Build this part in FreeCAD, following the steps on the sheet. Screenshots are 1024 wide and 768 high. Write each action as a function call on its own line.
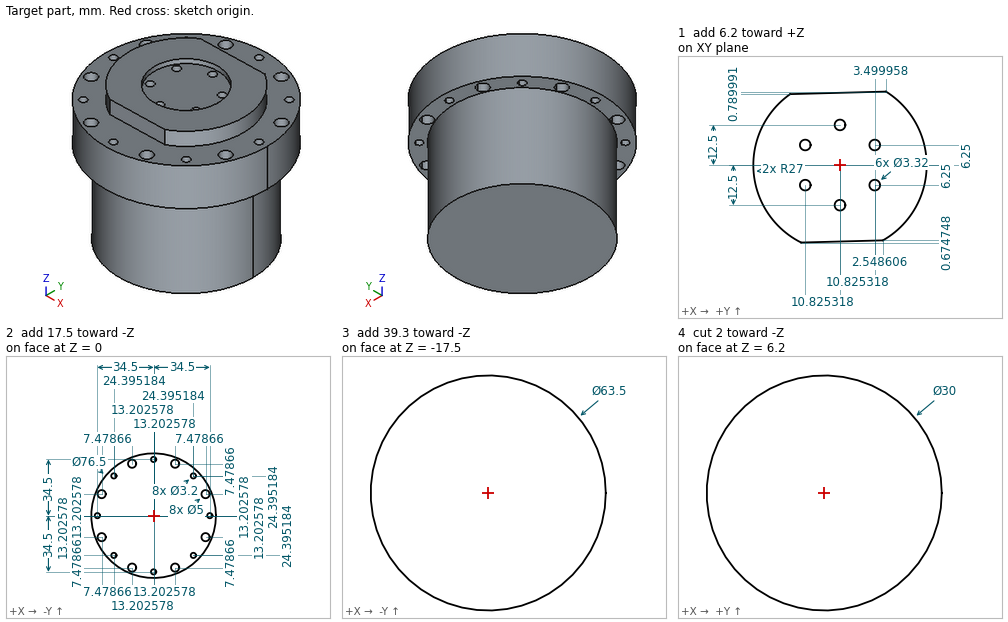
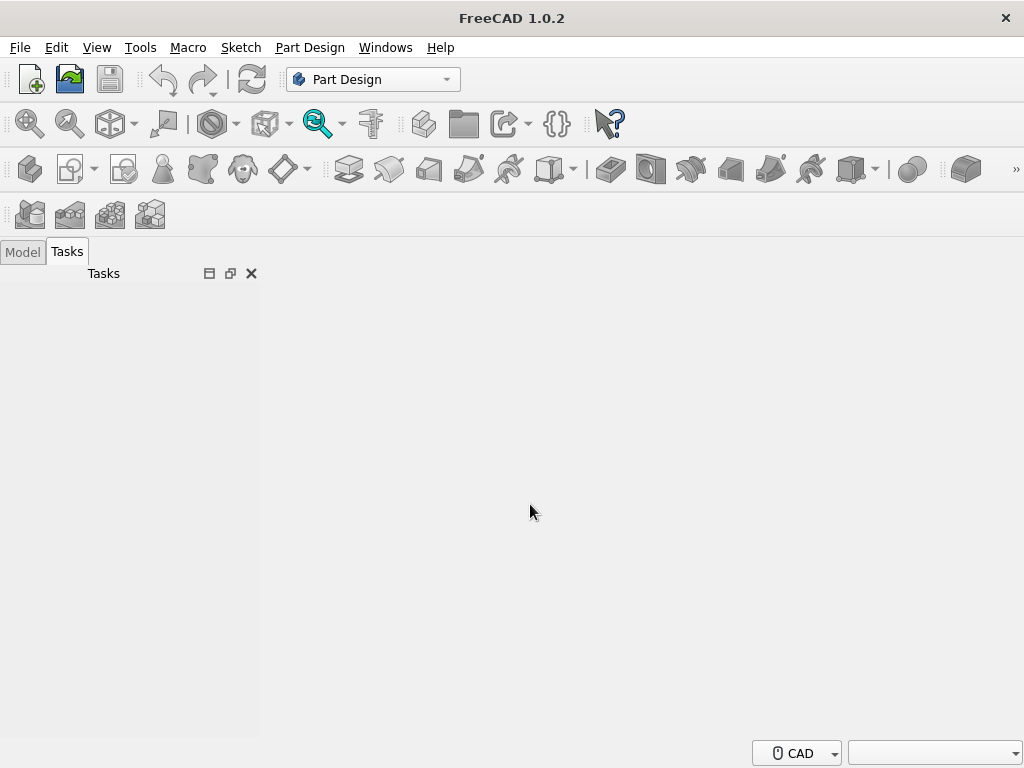
key(ctrl+n)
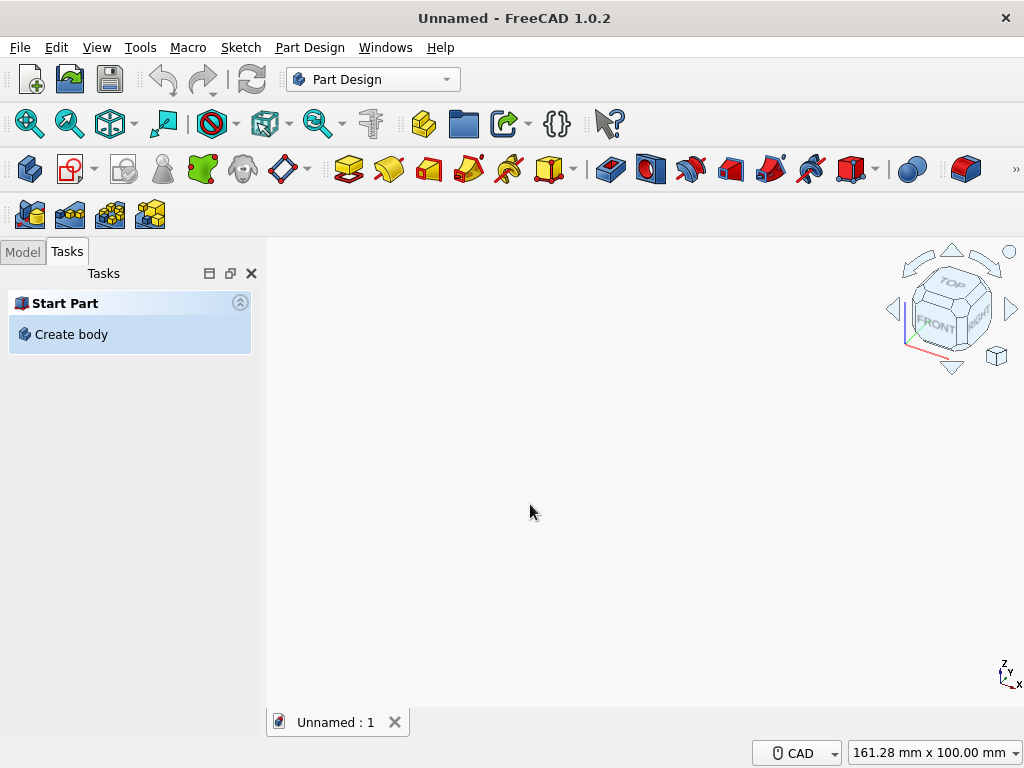
click(70, 170)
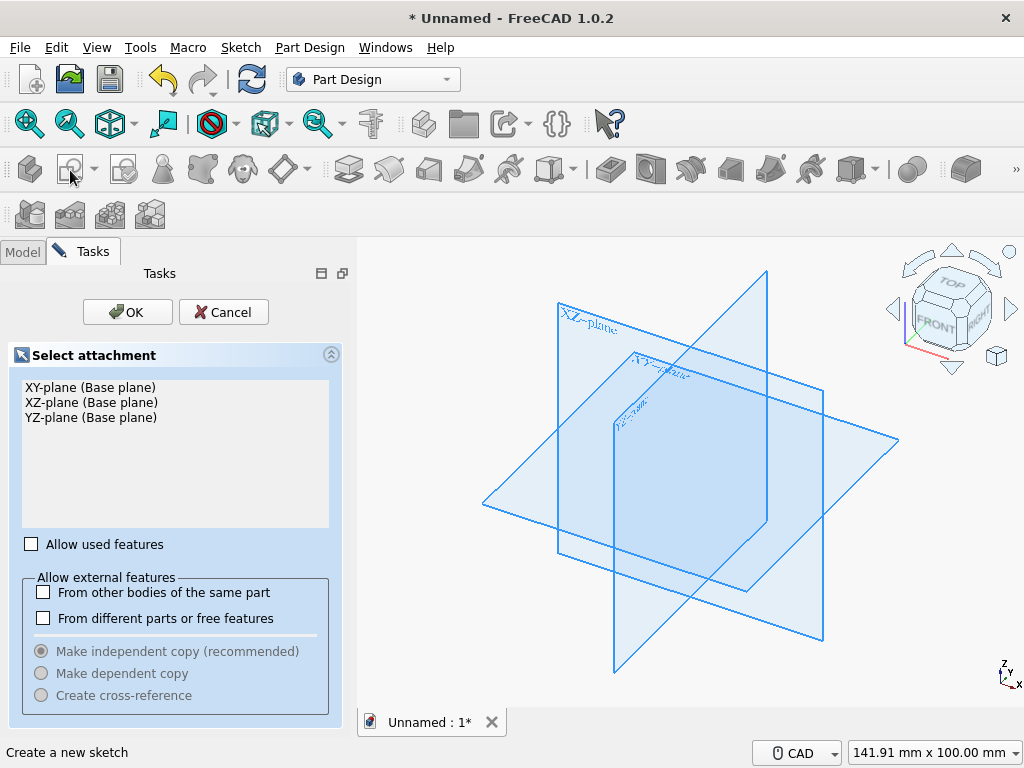
click(82, 388)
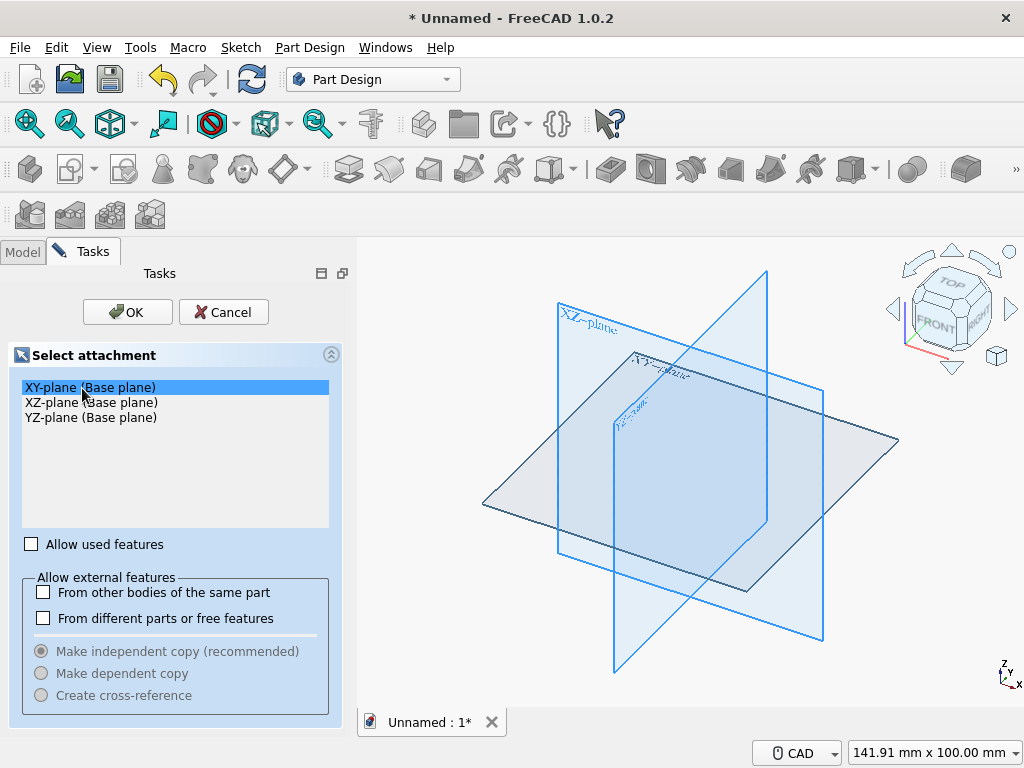
click(128, 312)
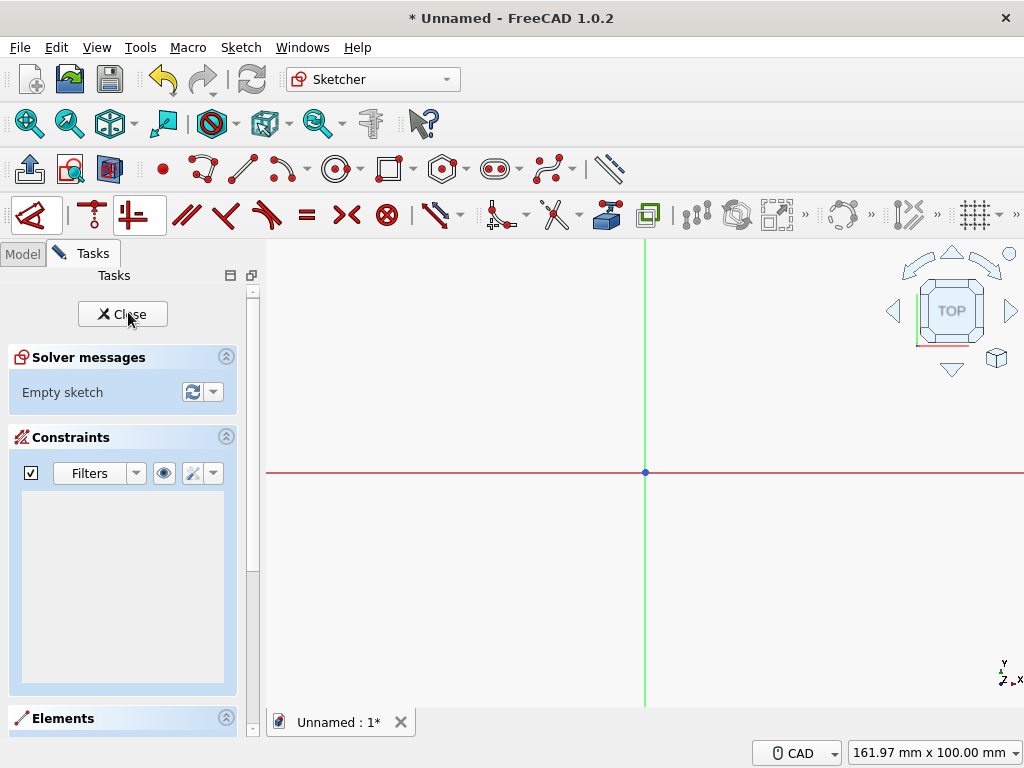
click(244, 170)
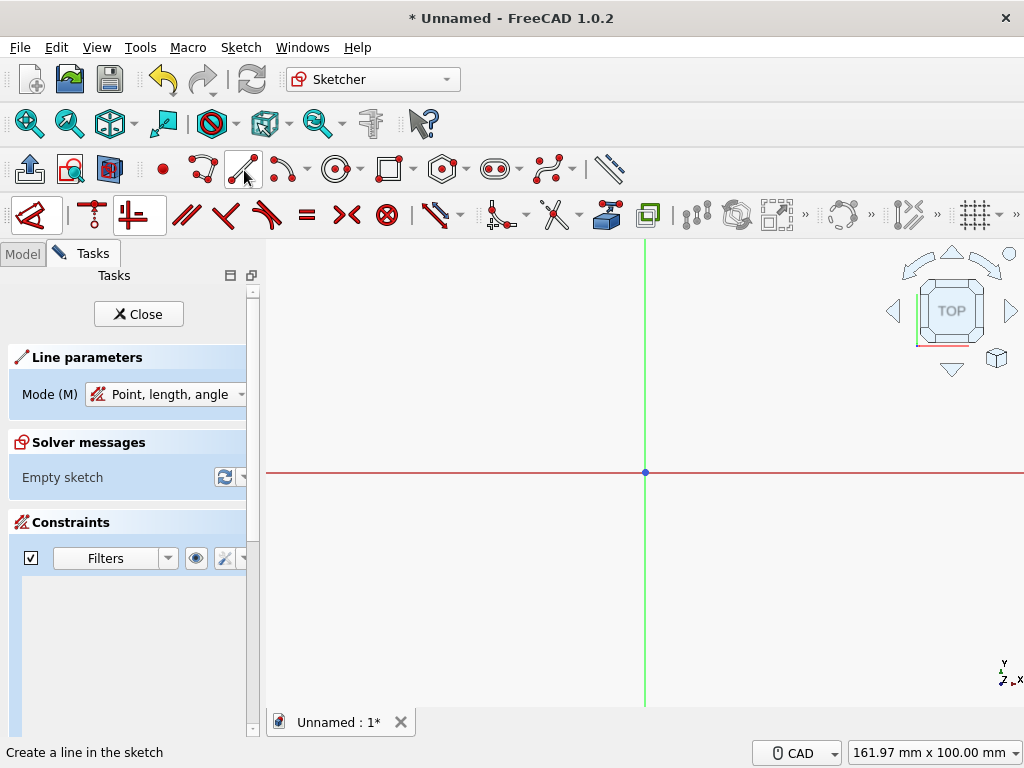
click(712, 366)
click(572, 374)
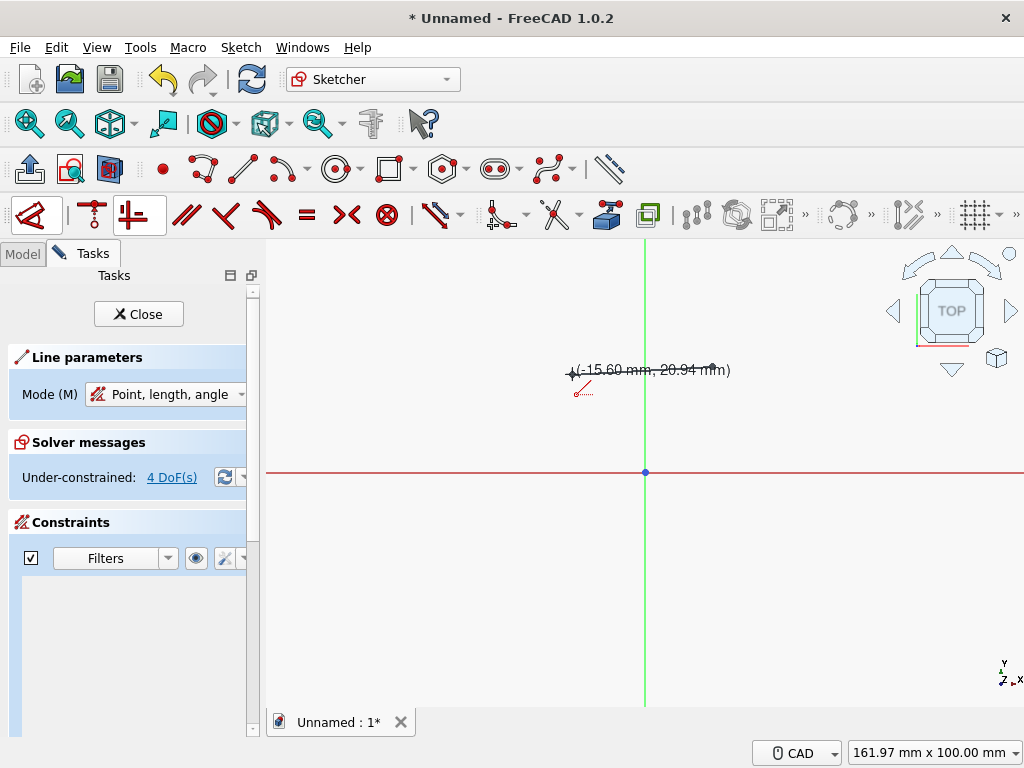
click(588, 586)
click(708, 579)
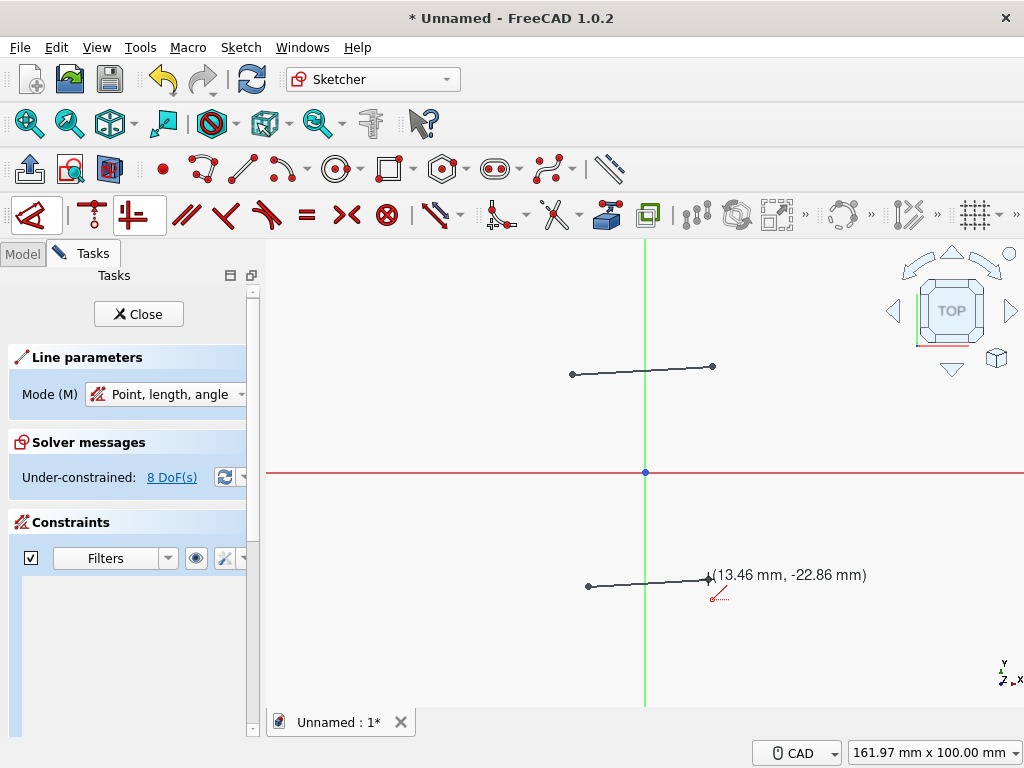
click(310, 170)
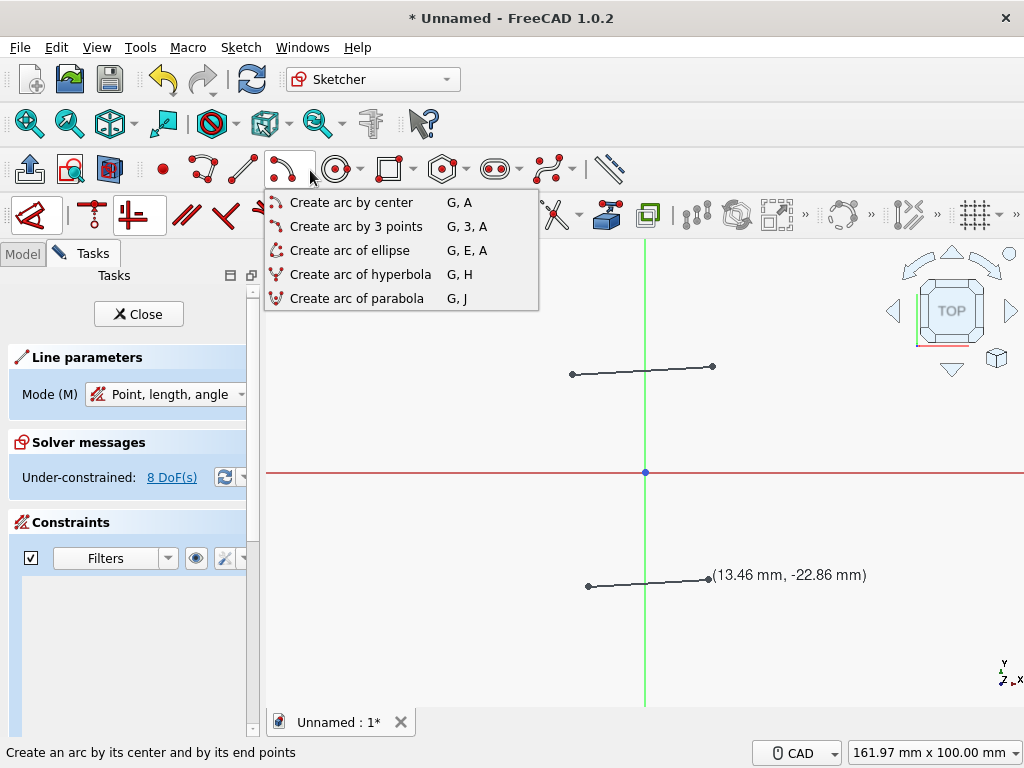
click(402, 226)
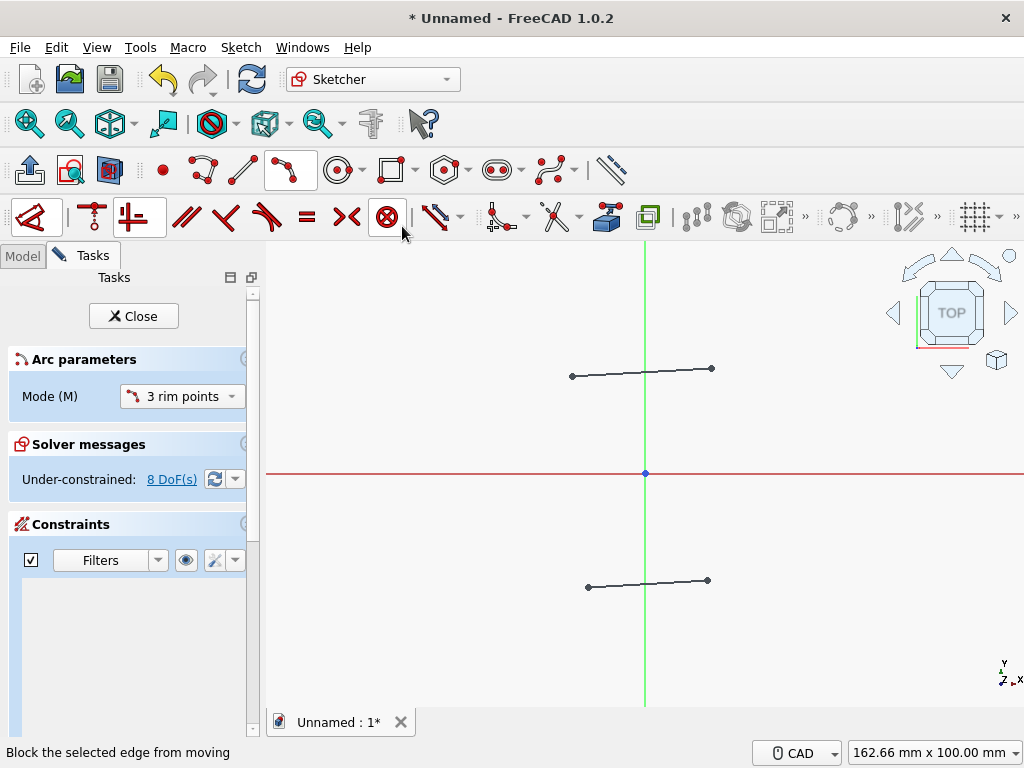
click(572, 376)
click(588, 588)
click(520, 457)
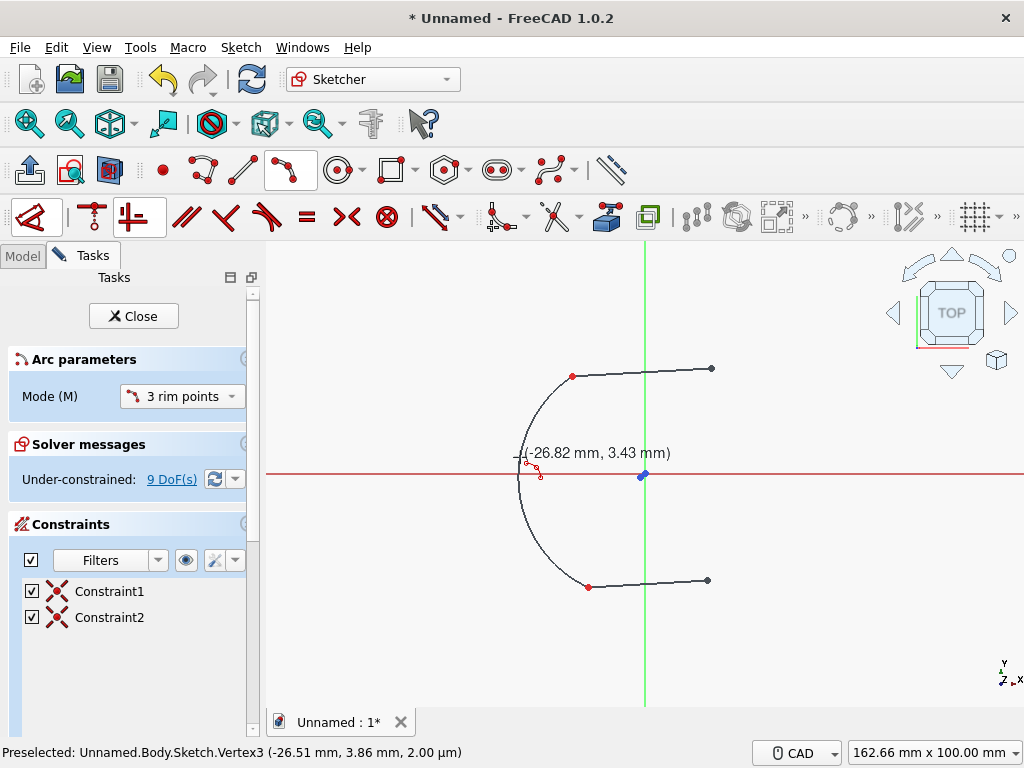
click(708, 581)
click(712, 368)
click(768, 502)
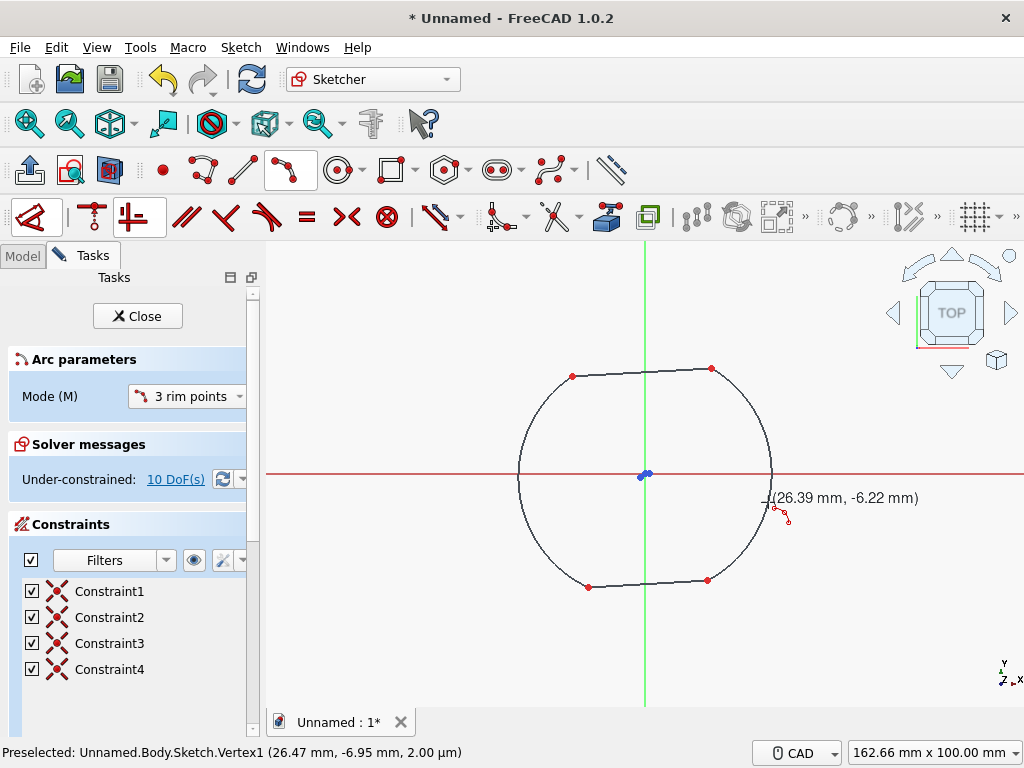
click(338, 170)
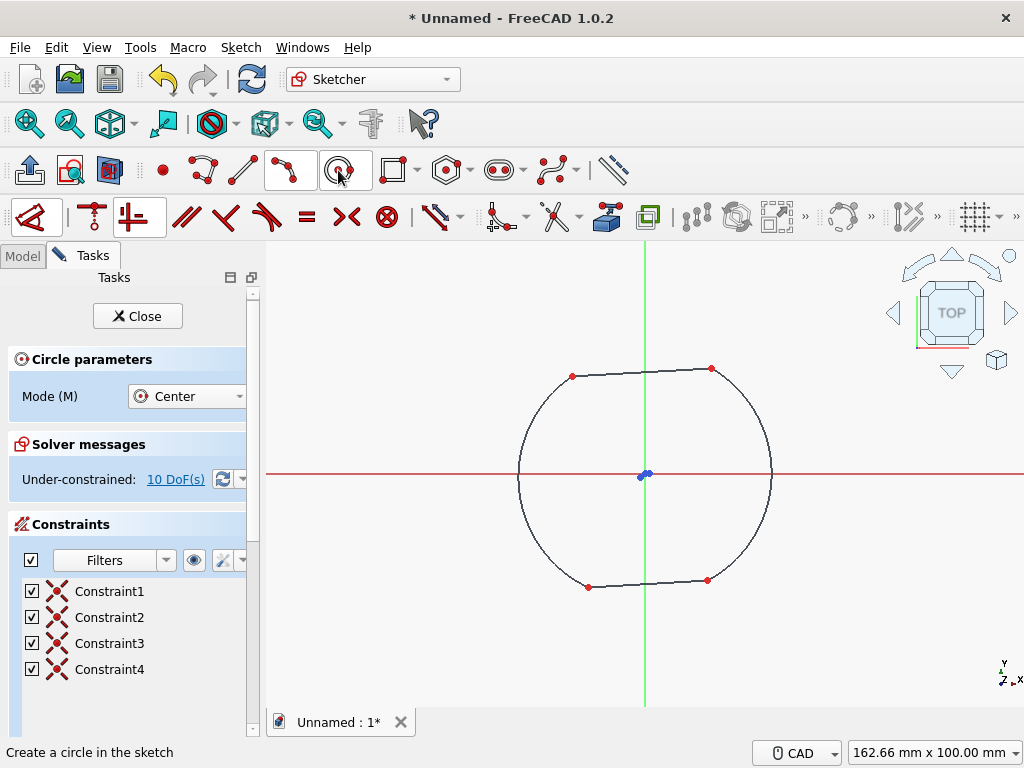
scroll(645, 532, up, 6)